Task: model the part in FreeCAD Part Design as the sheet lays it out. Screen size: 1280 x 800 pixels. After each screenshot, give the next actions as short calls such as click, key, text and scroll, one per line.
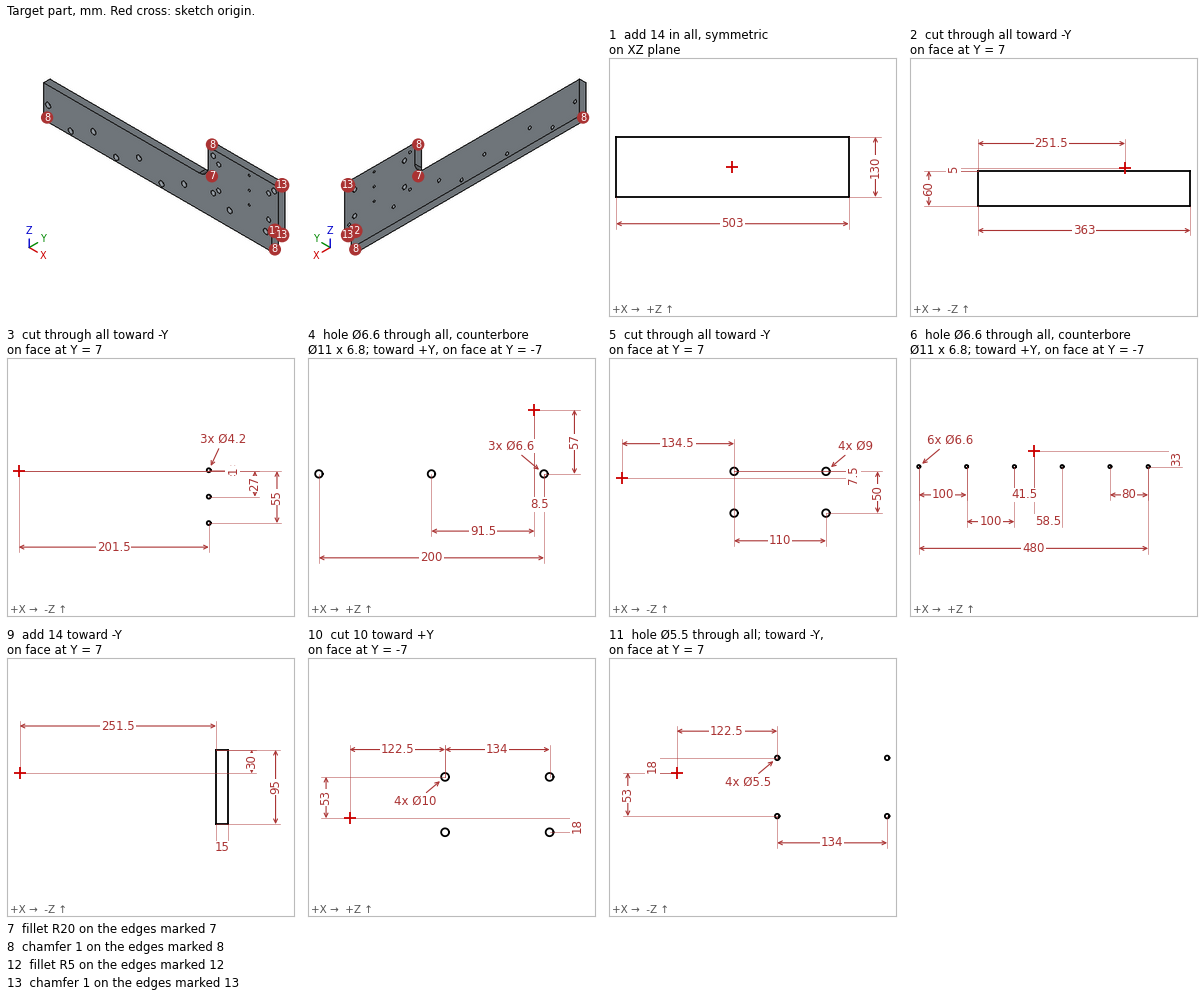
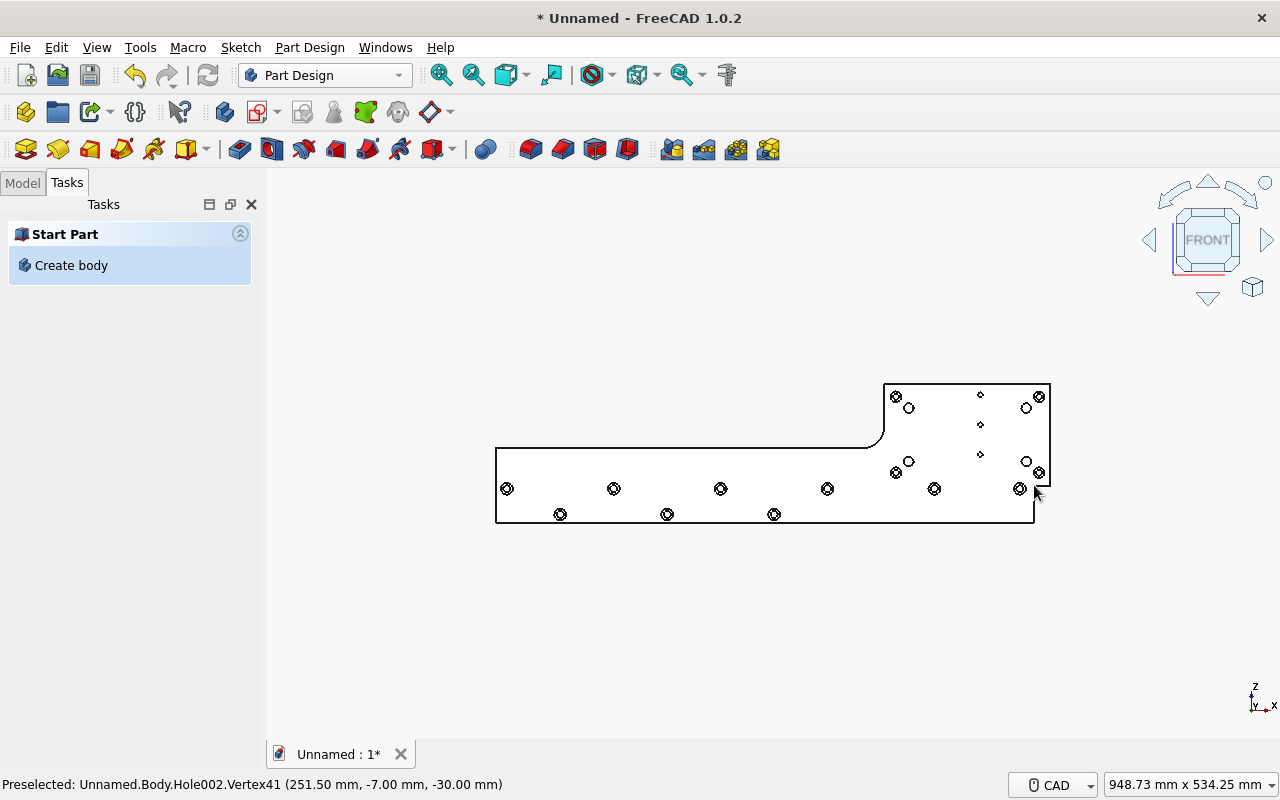
key(3)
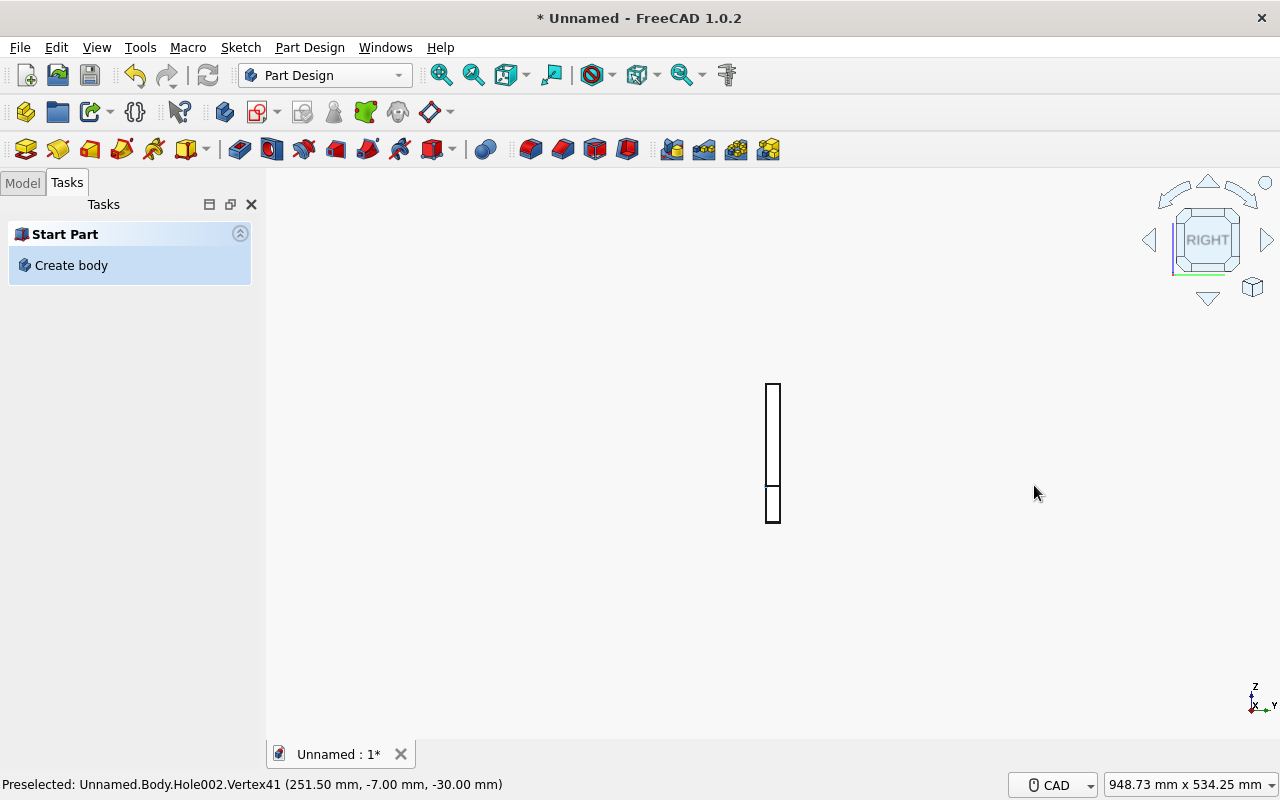
key(v)
key(f)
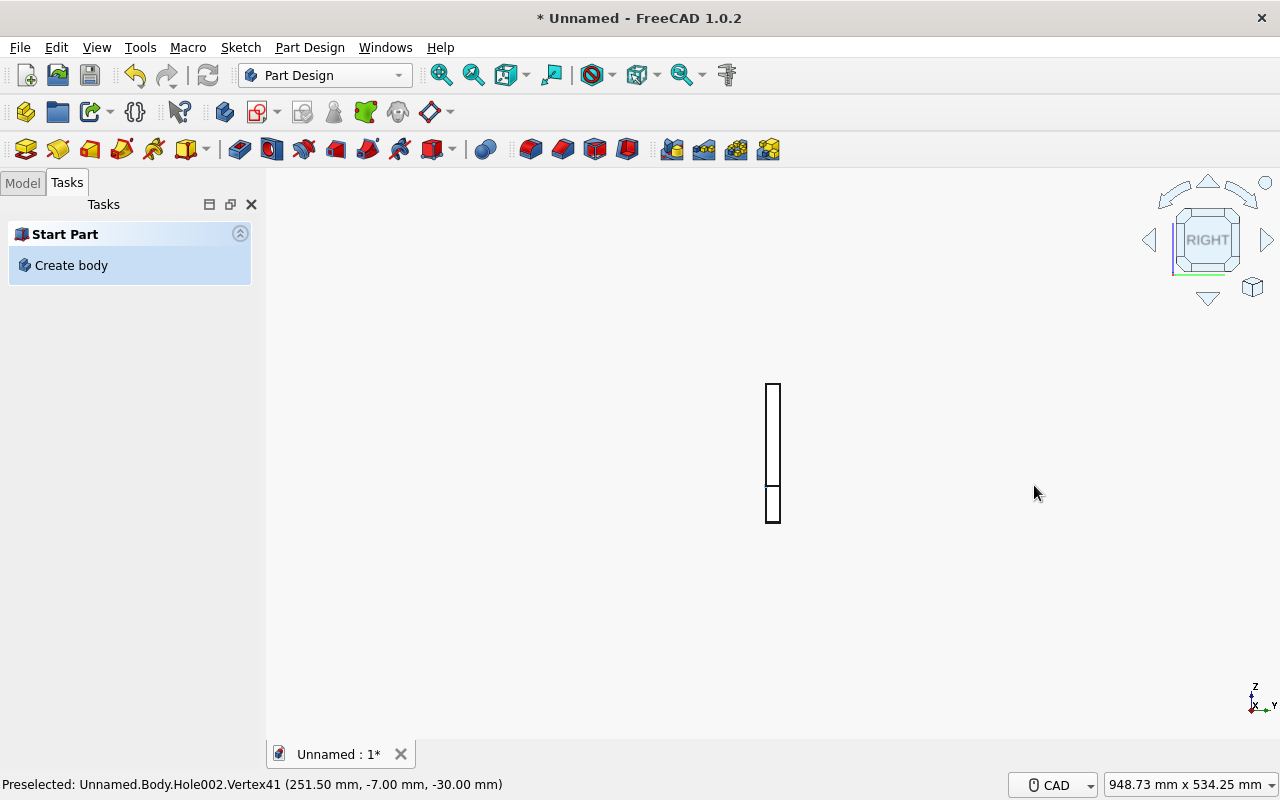
scroll(773, 485, up, 5)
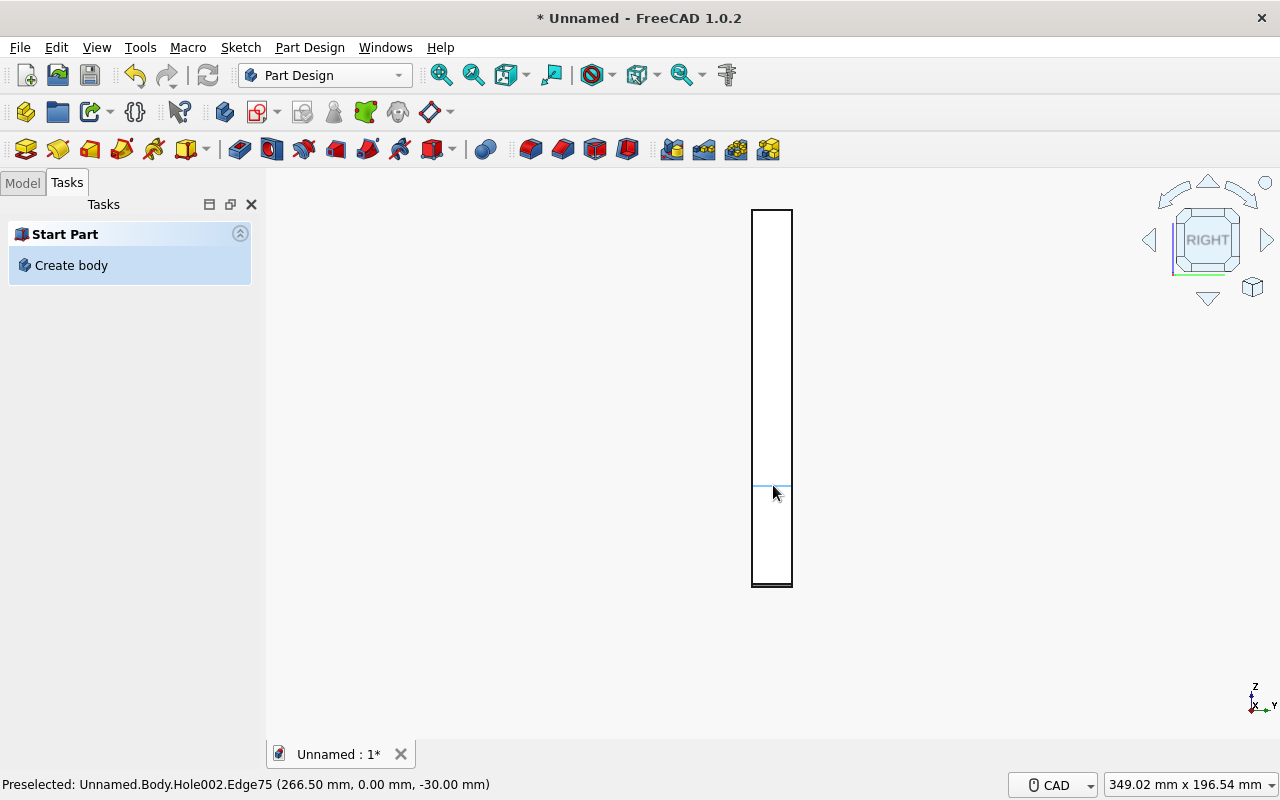
click(442, 76)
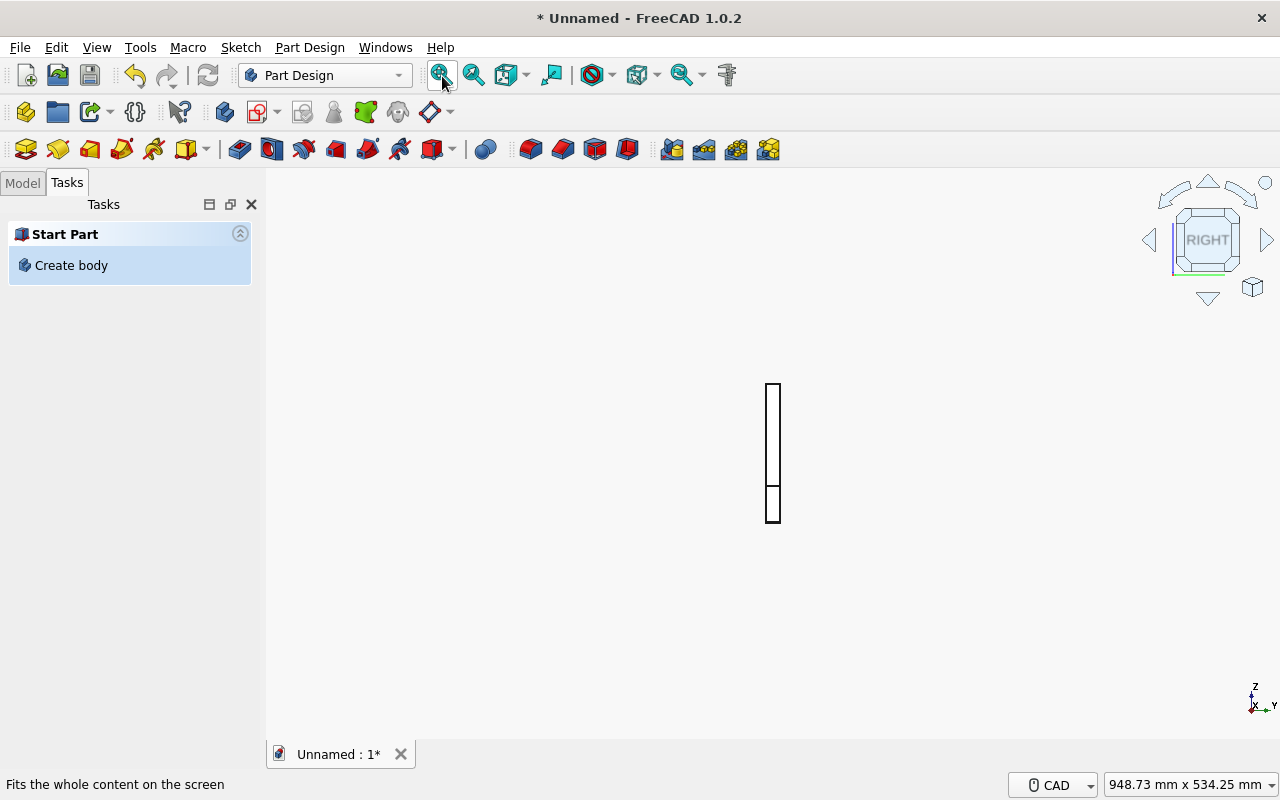
key(5)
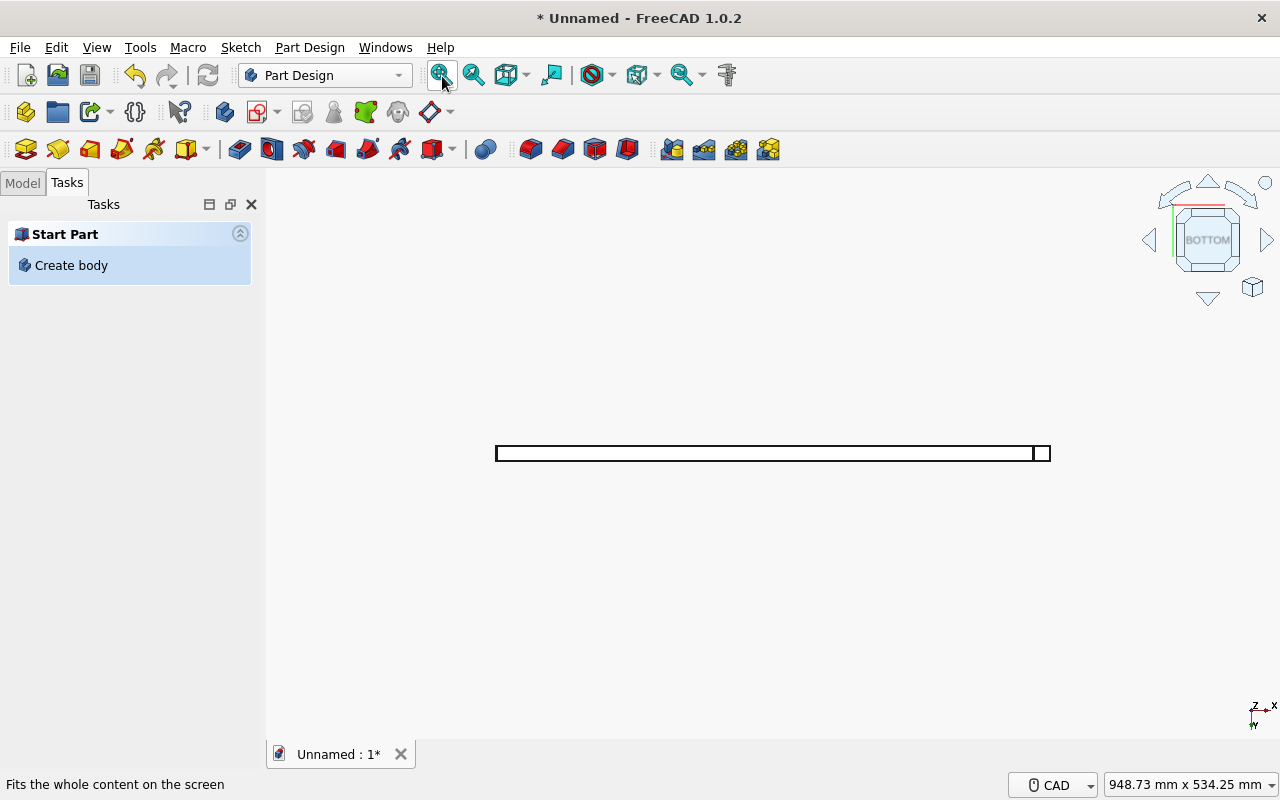
scroll(1034, 452, up, 5)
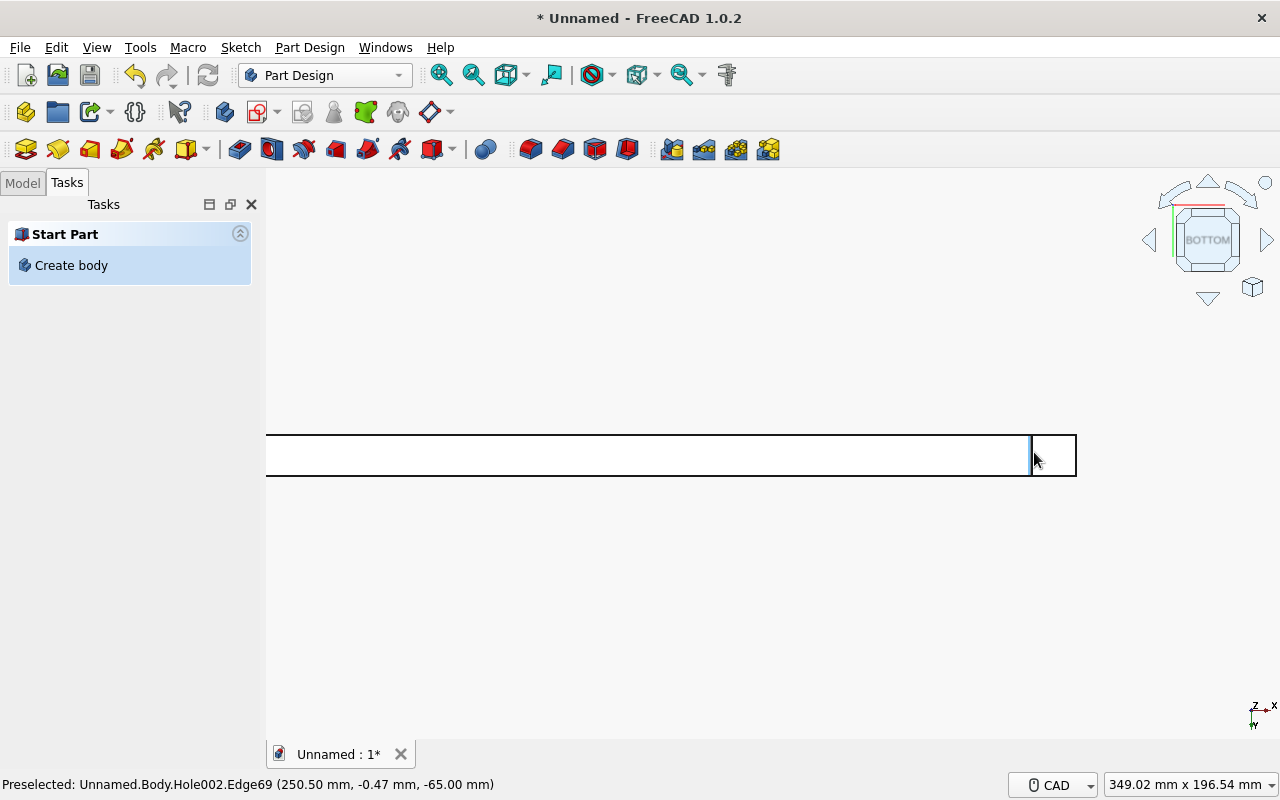
key(v)
key(f)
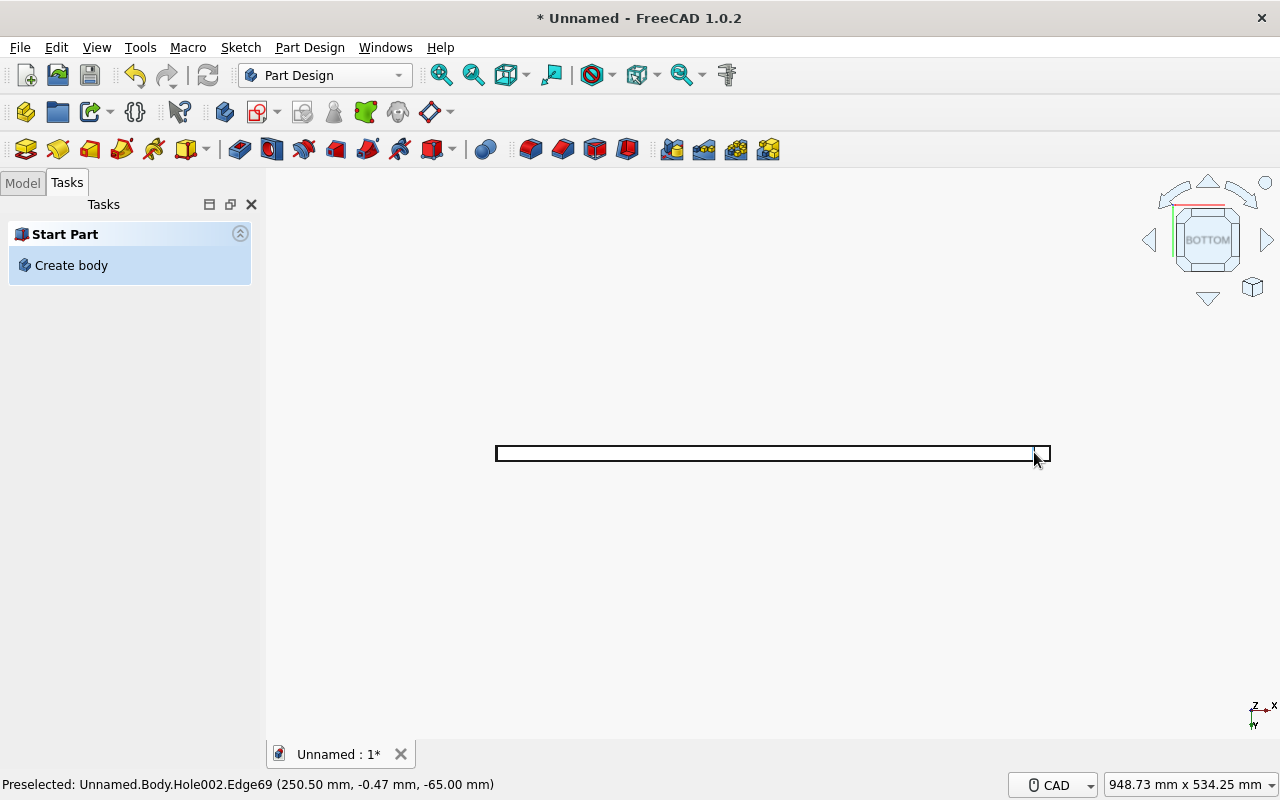
key(4)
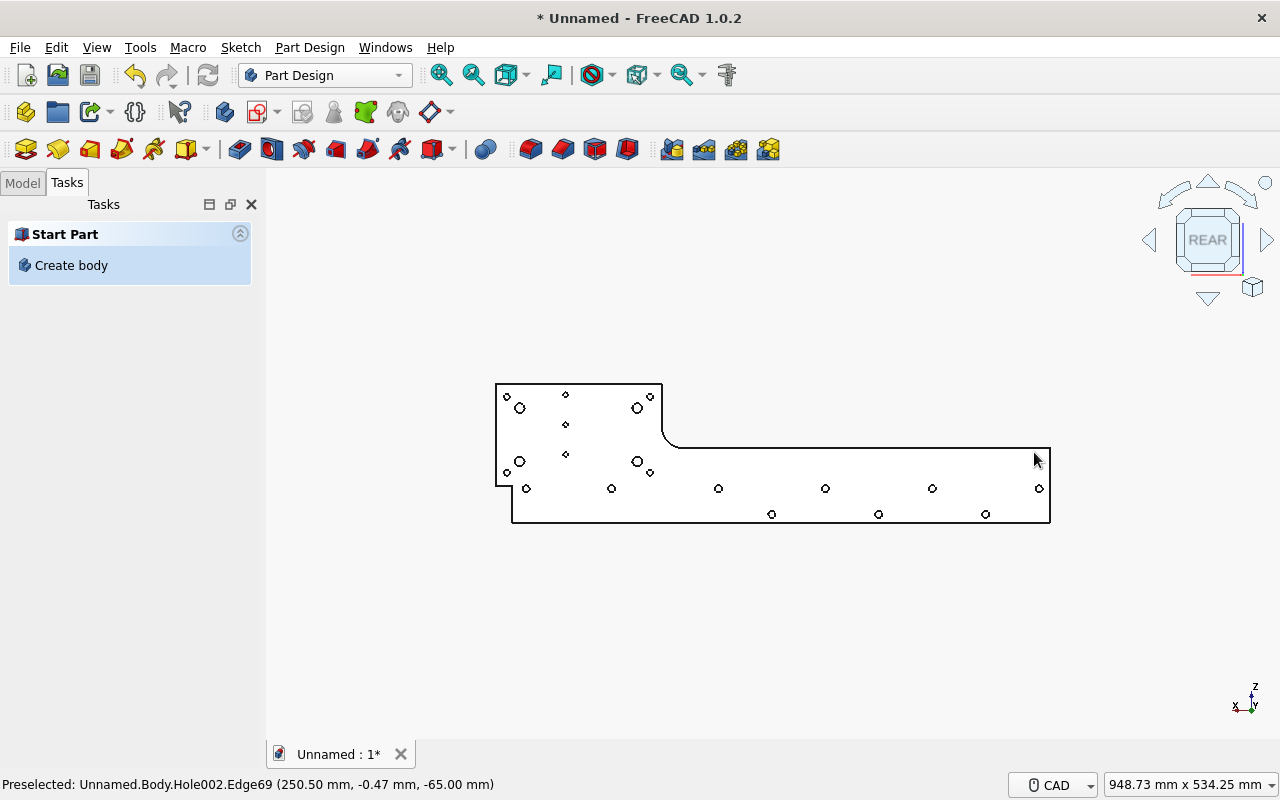
scroll(512, 485, up, 5)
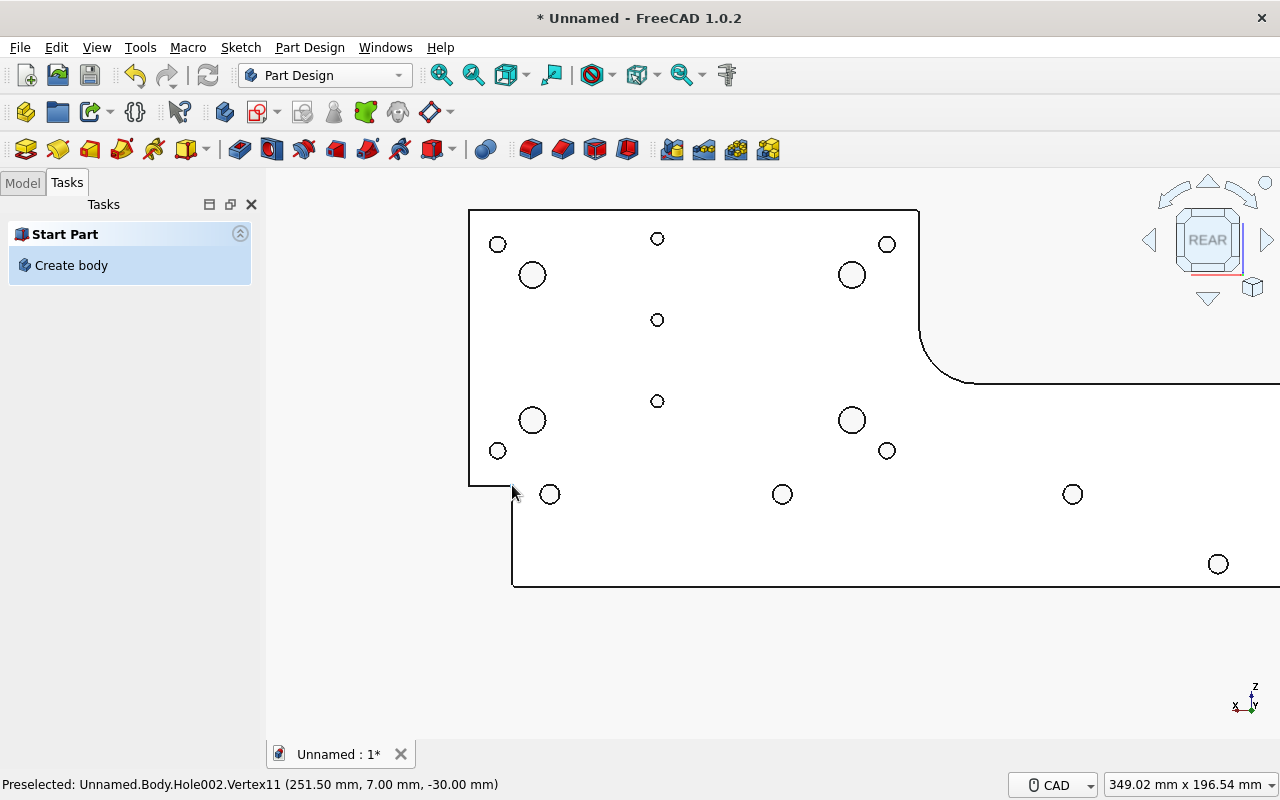
key(v)
key(f)